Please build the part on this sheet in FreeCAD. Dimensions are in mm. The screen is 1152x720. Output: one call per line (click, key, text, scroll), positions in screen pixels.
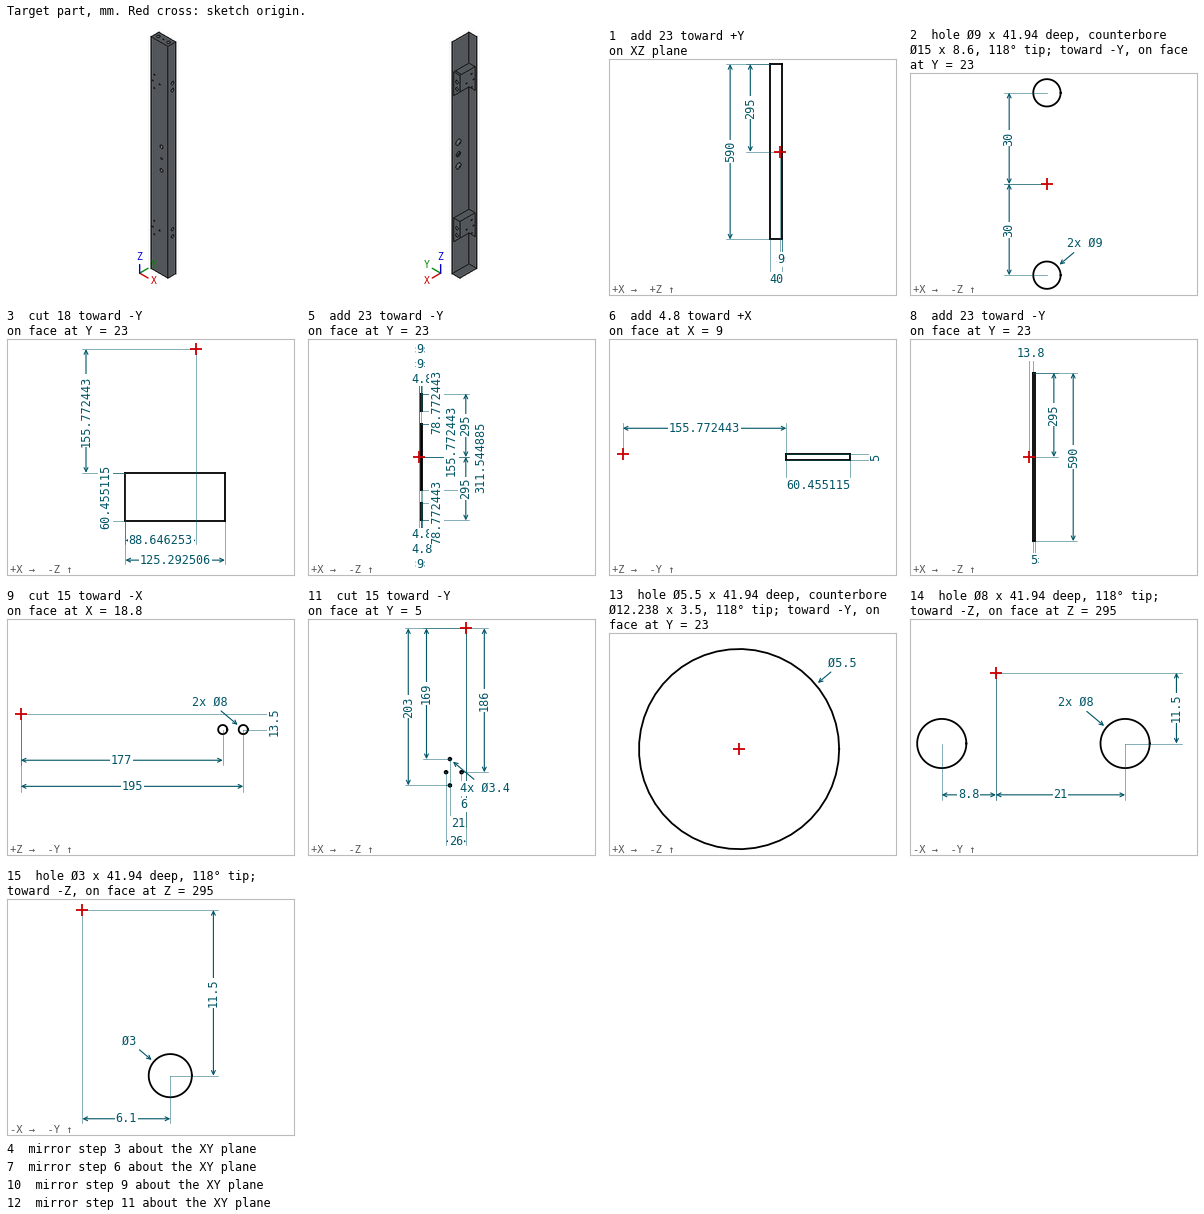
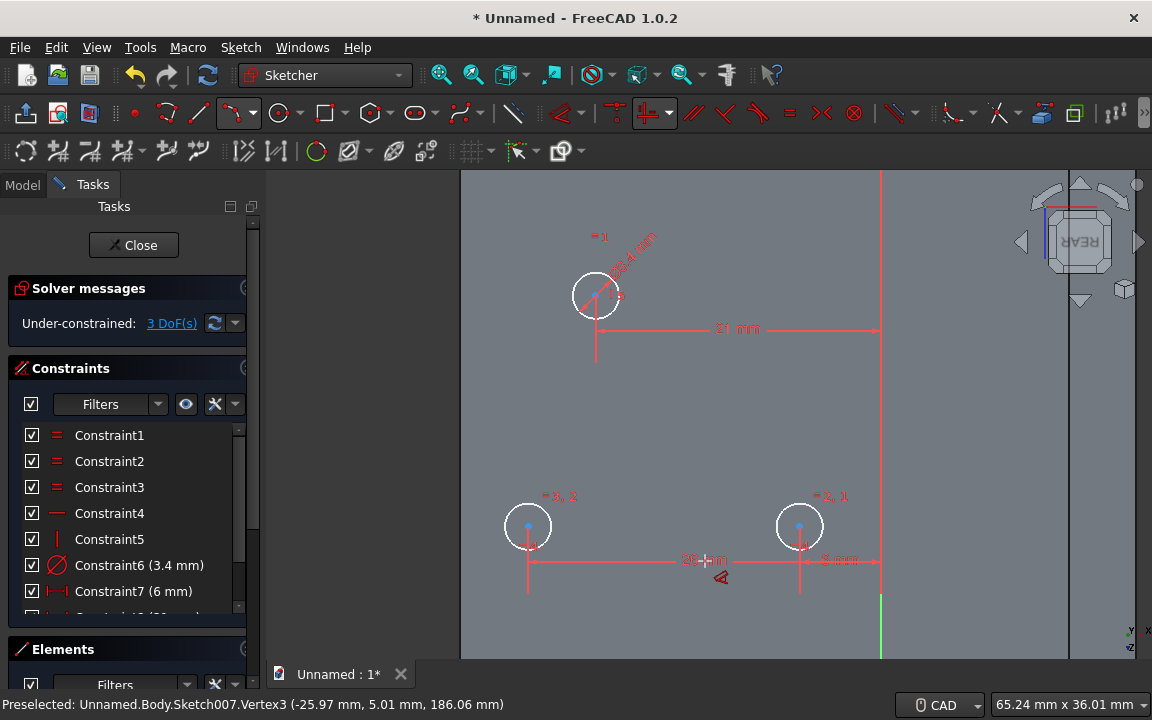
click(596, 296)
click(915, 247)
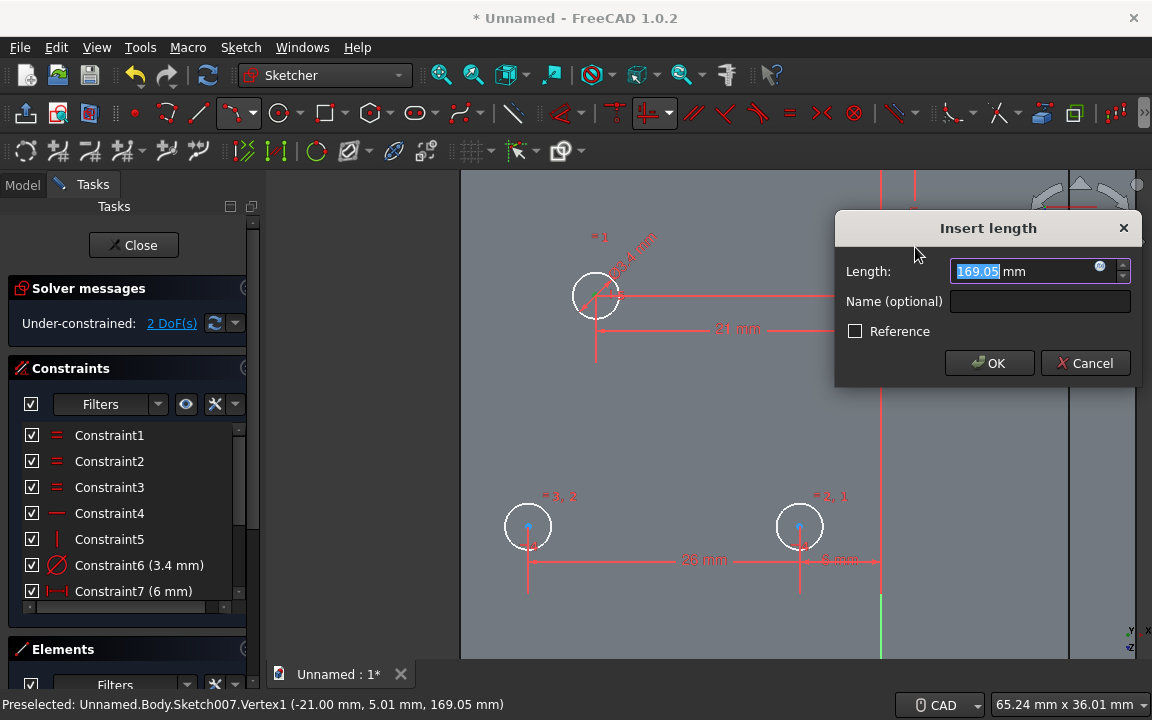
text(169)
key(Return)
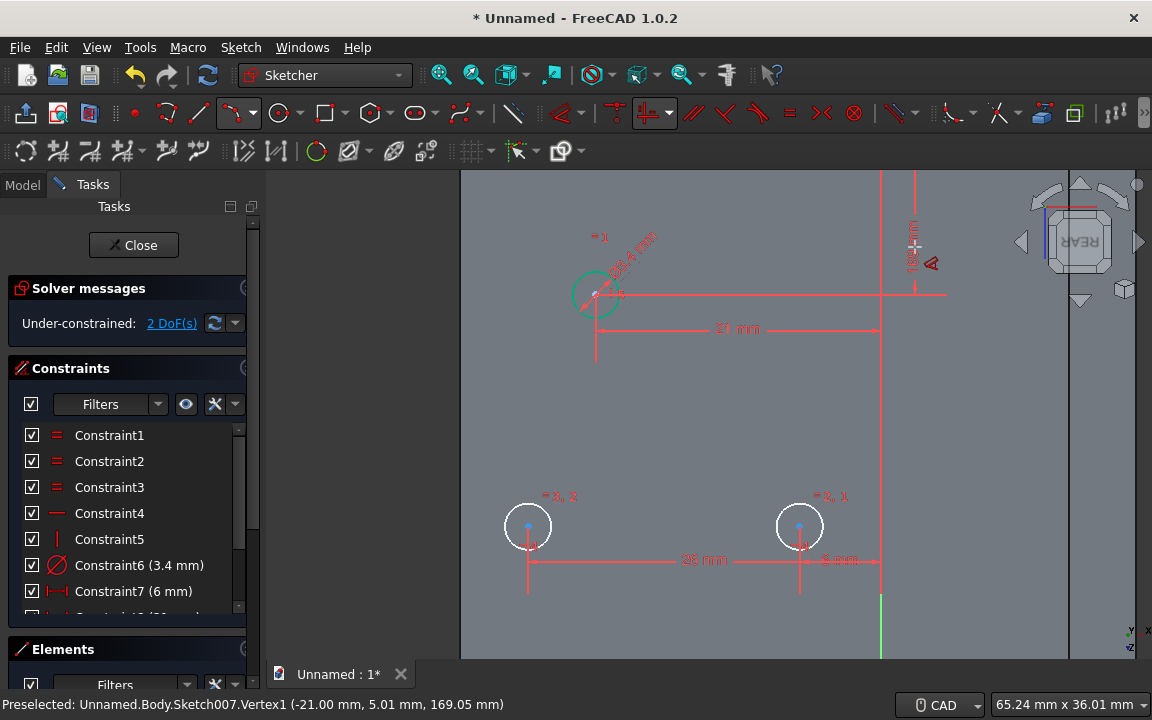
click(800, 527)
click(915, 362)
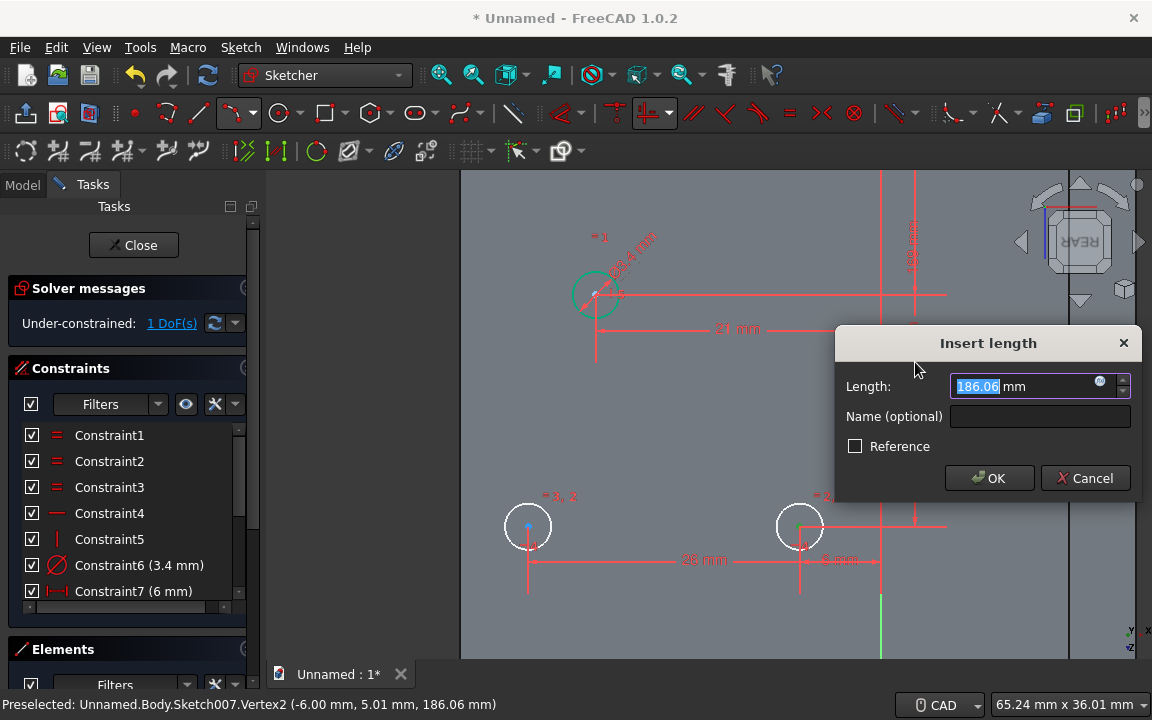
text(186)
key(Return)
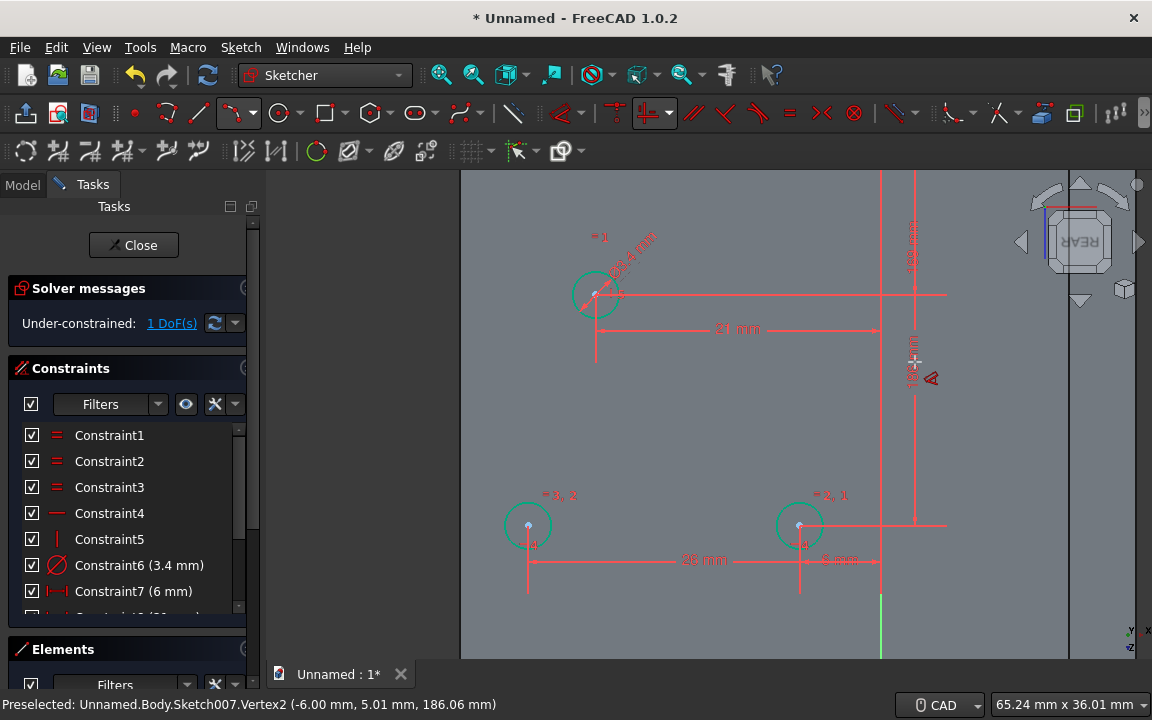
scroll(612, 279, down, 3)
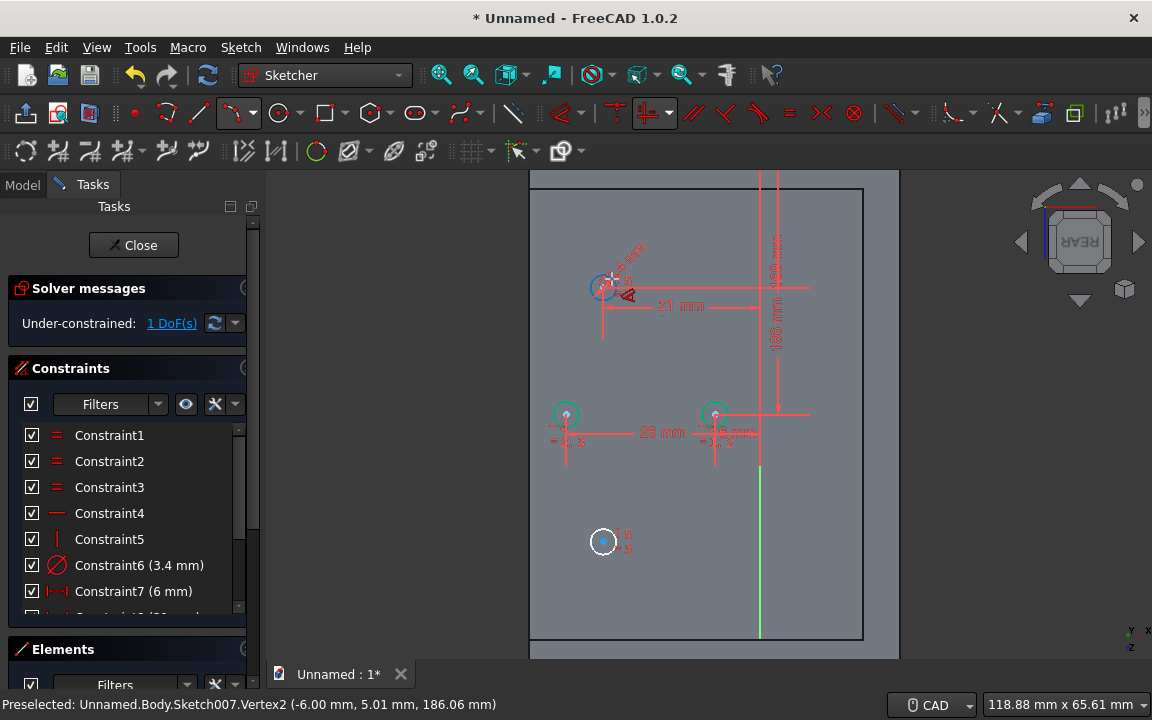
click(603, 542)
click(794, 370)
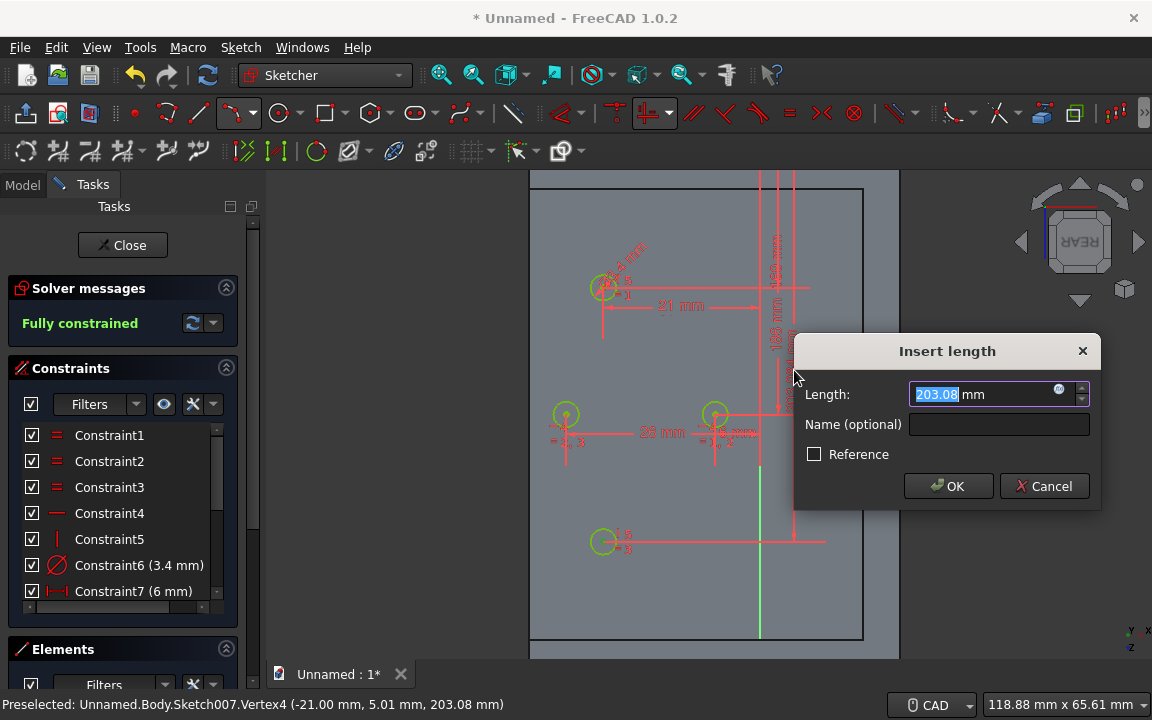
text(203)
key(Return)
key(Escape)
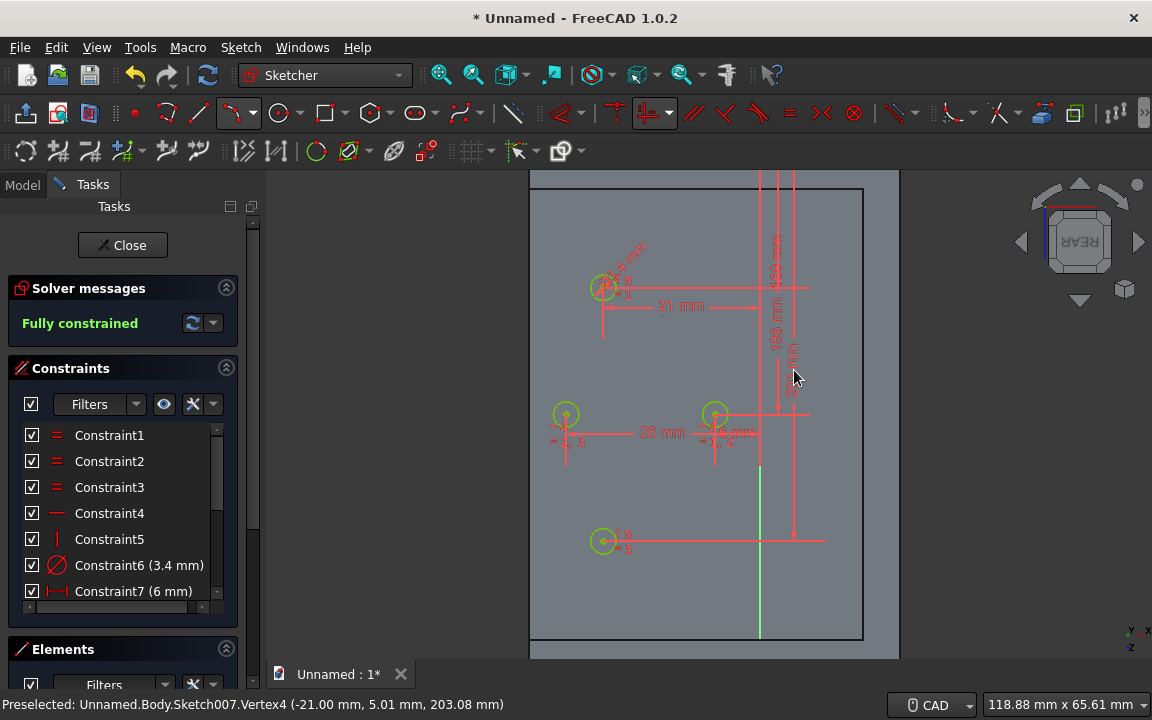
click(123, 245)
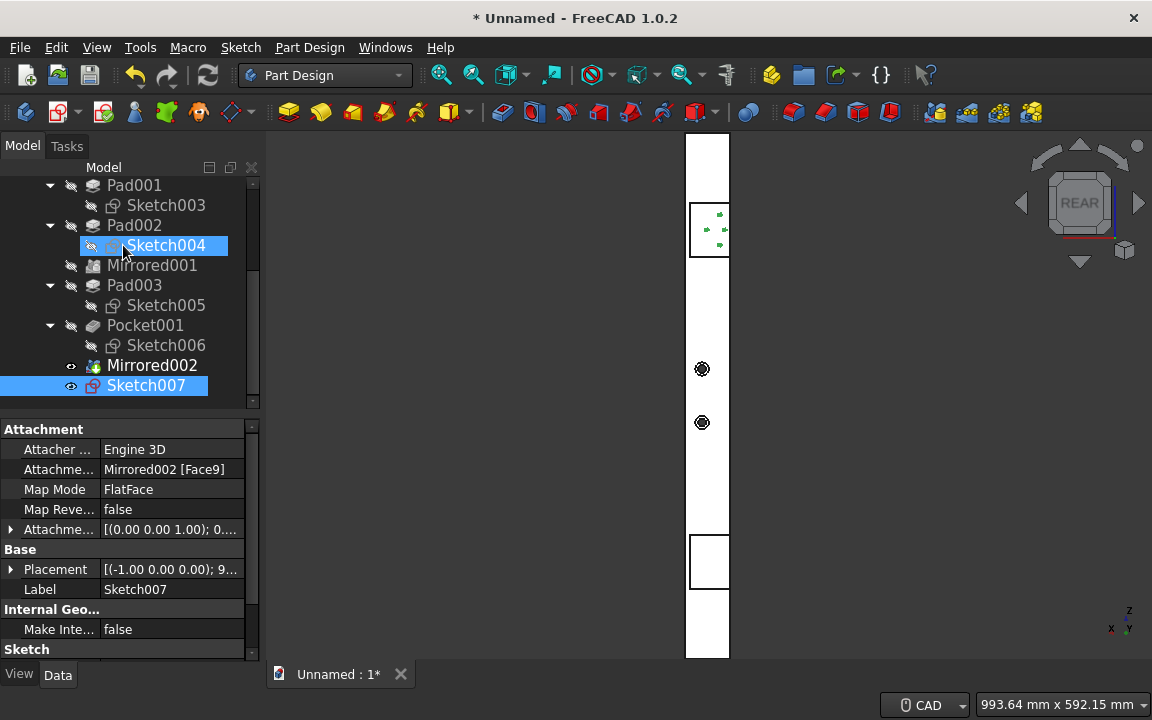
click(504, 112)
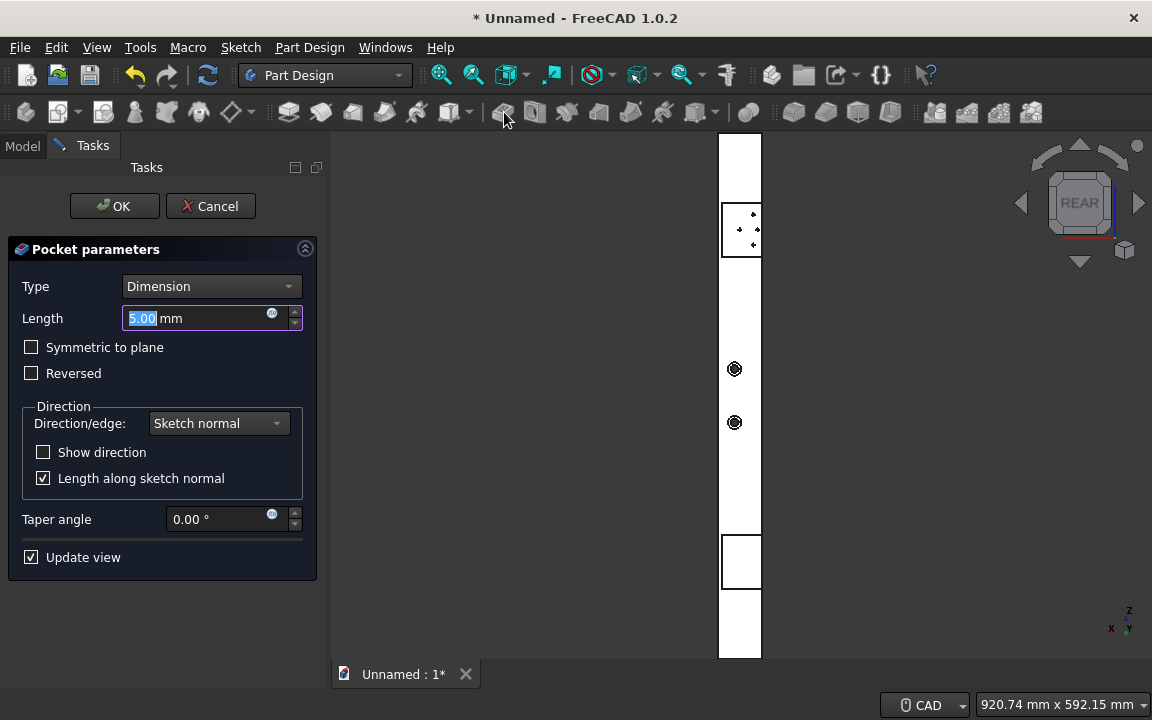
text(15)
key(Tab)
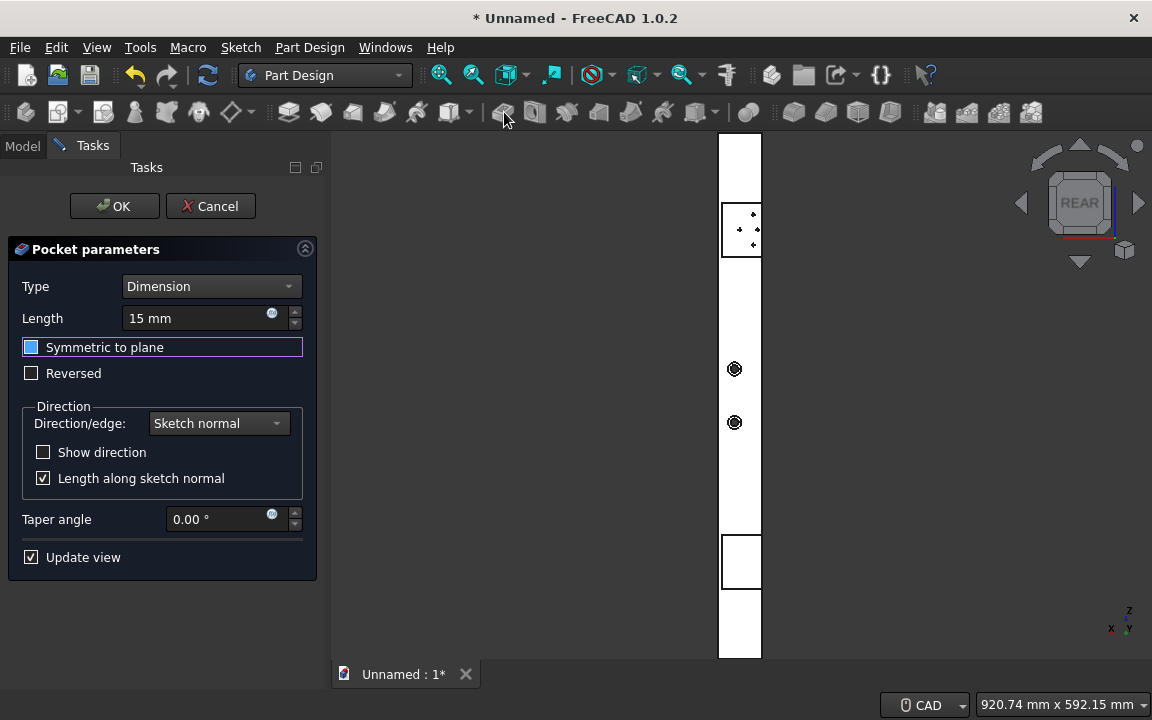
click(115, 206)